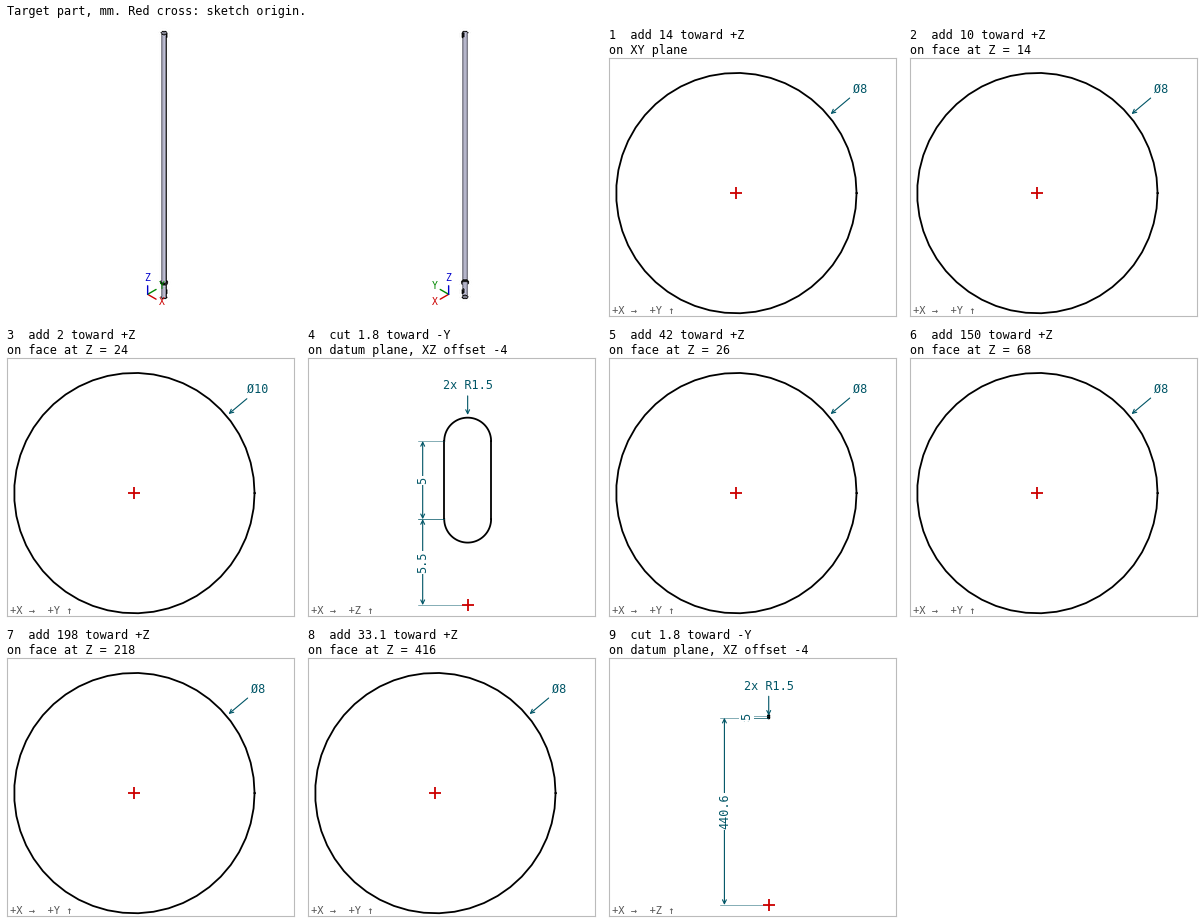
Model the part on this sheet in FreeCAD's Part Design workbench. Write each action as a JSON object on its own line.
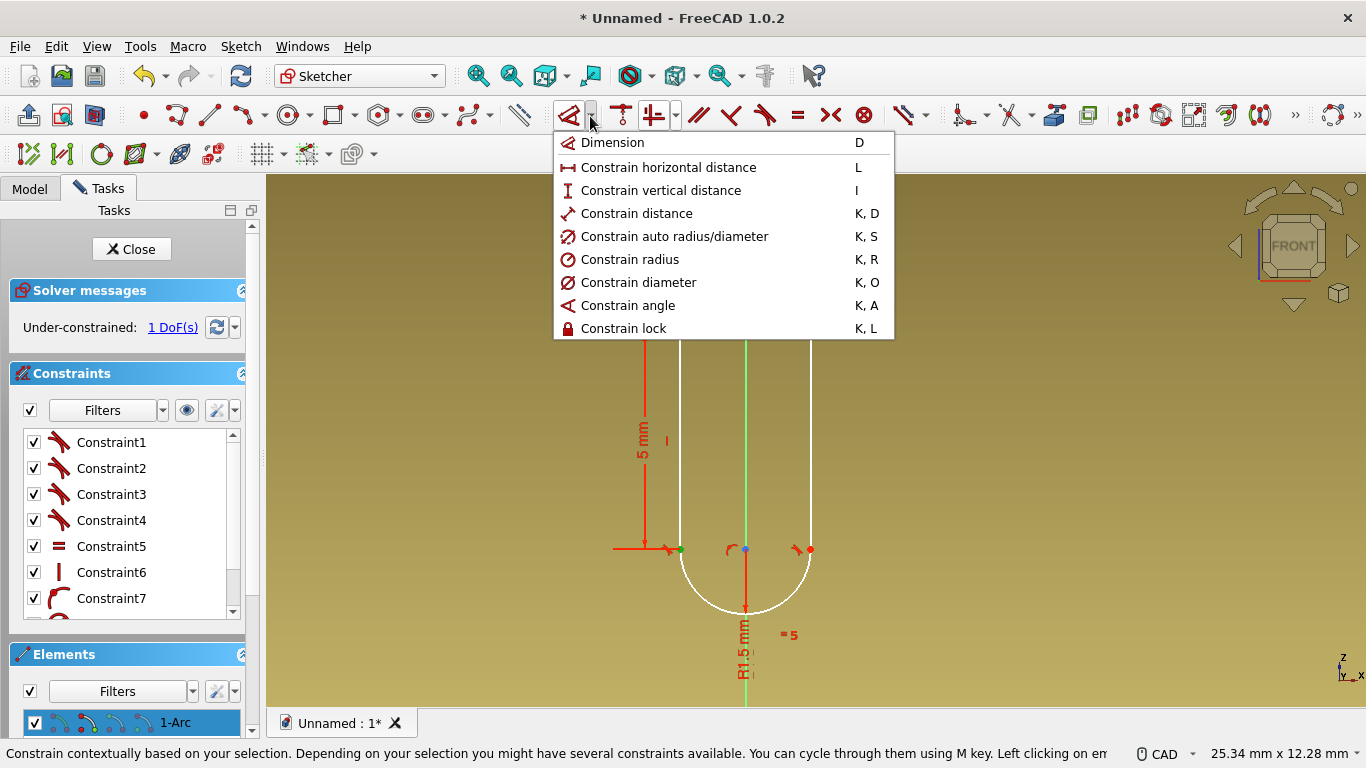
{"action": "left_click", "coordinate": [724, 190]}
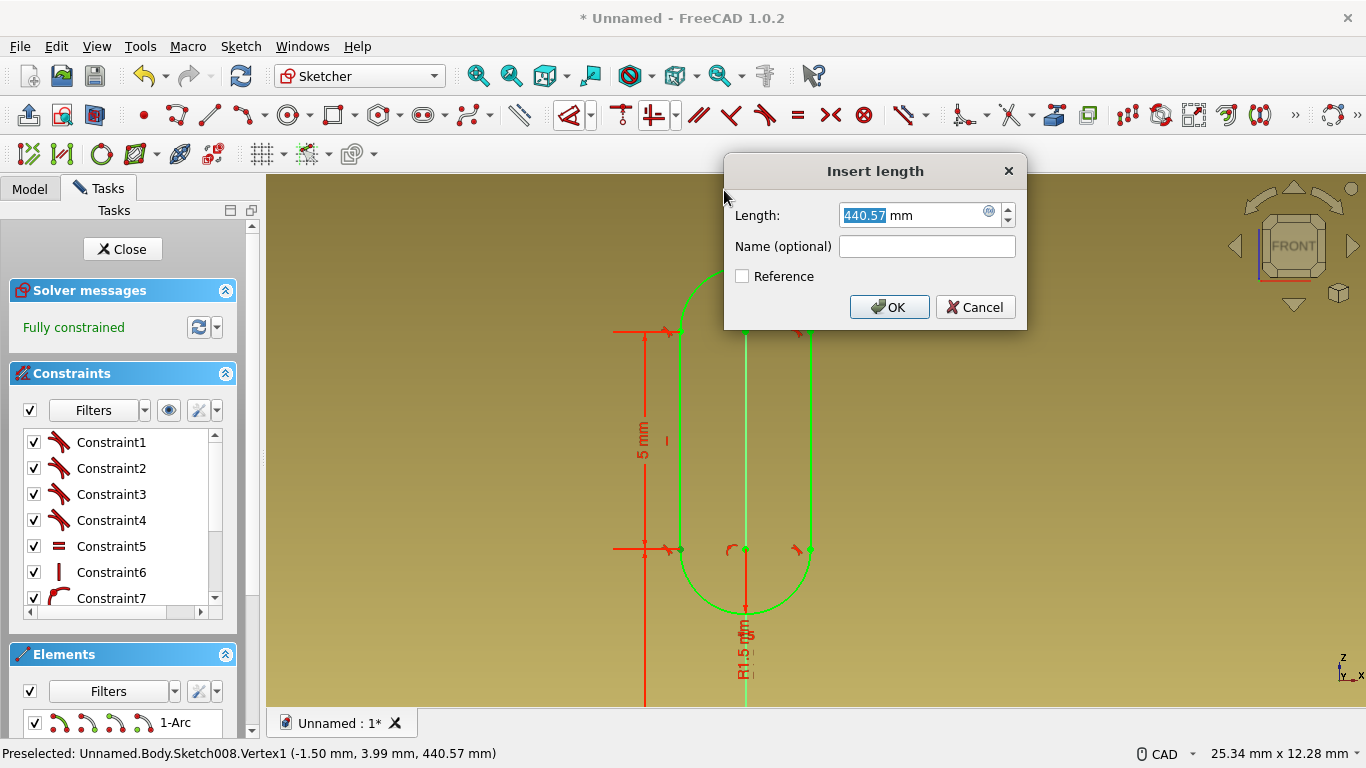
{"action": "type", "text": "440.6"}
{"action": "key", "text": "Return"}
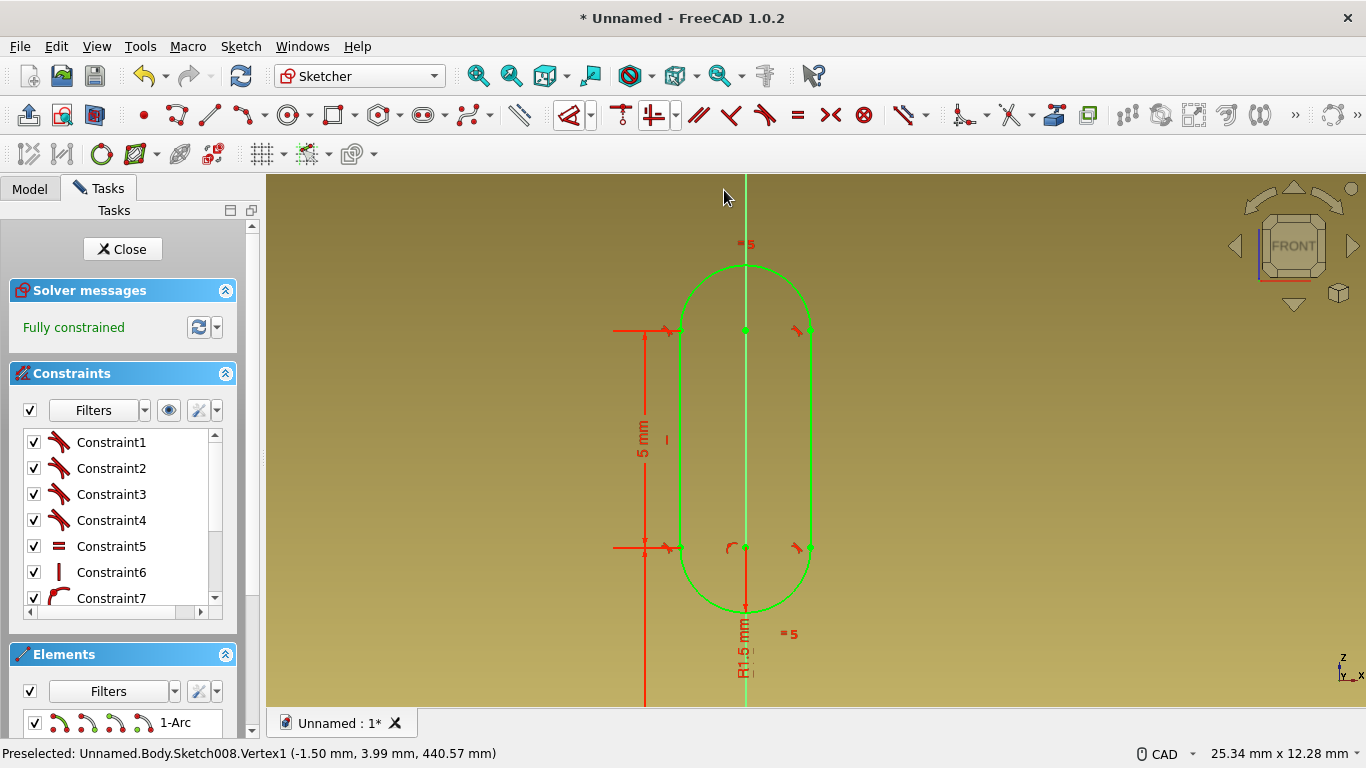
{"action": "left_click", "coordinate": [123, 249]}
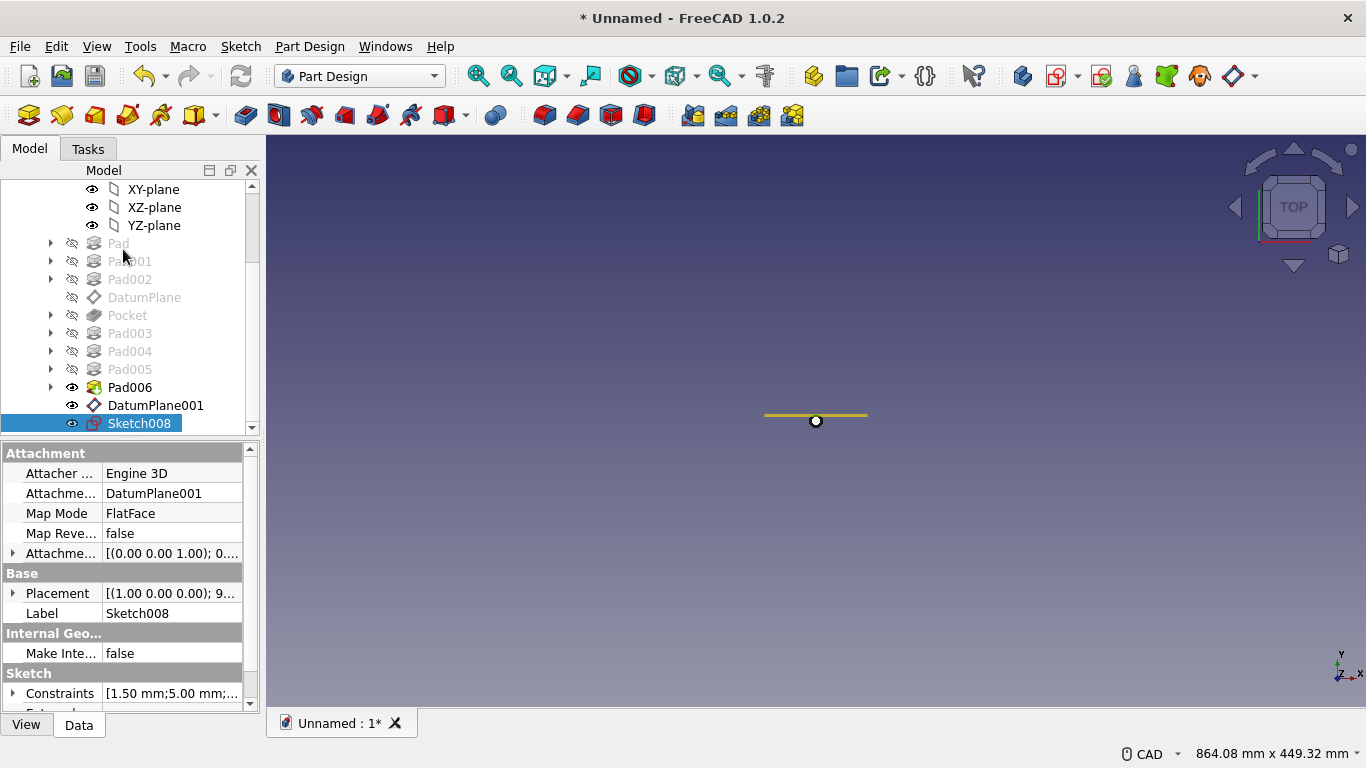
{"action": "left_click", "coordinate": [246, 116]}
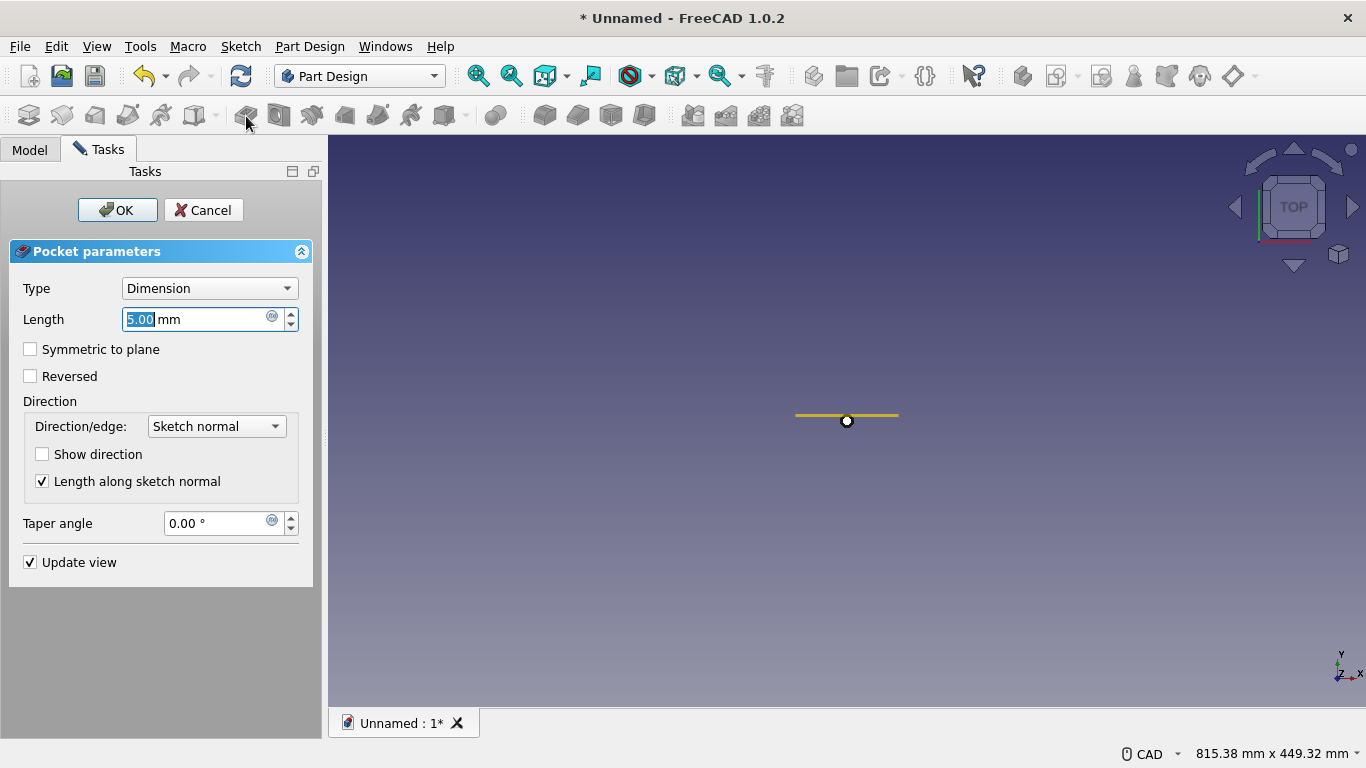
{"action": "type", "text": "1.8"}
{"action": "key", "text": "Tab"}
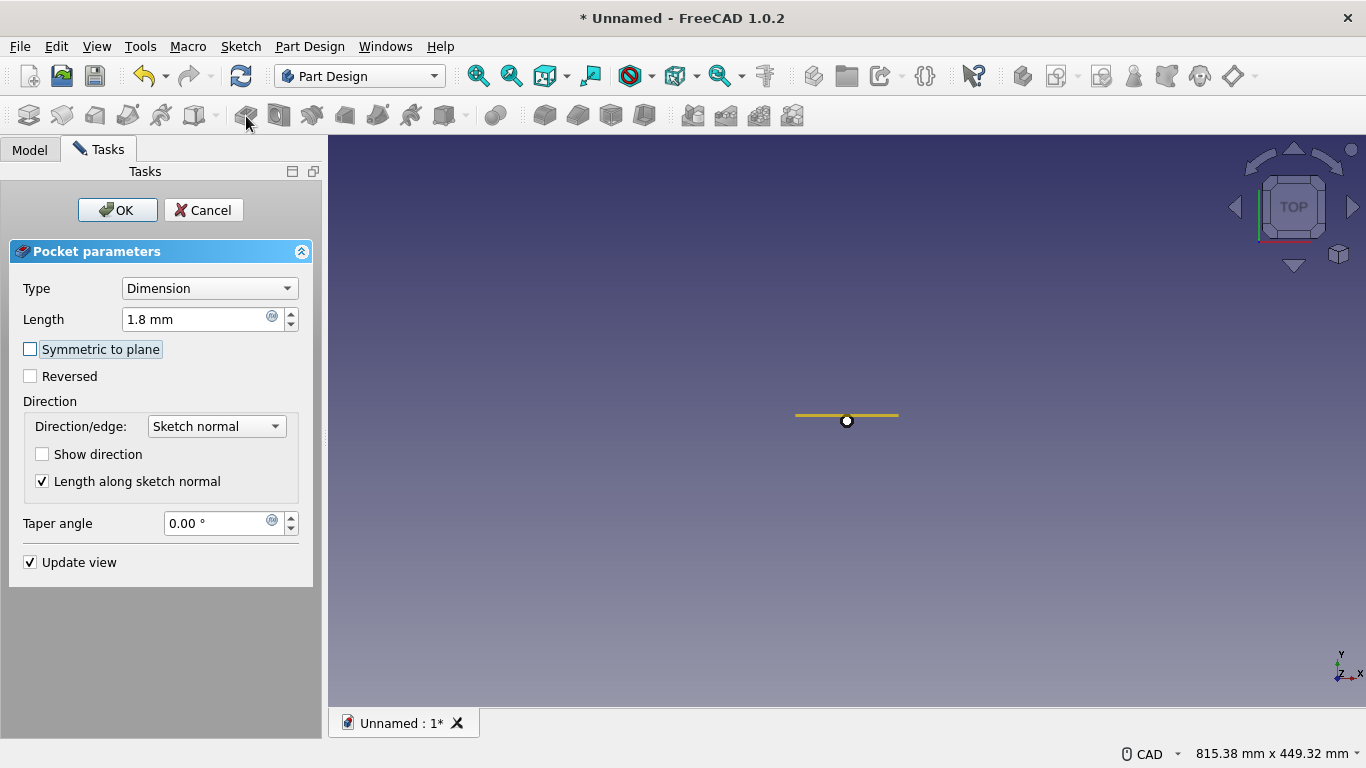
{"action": "left_click", "coordinate": [31, 376]}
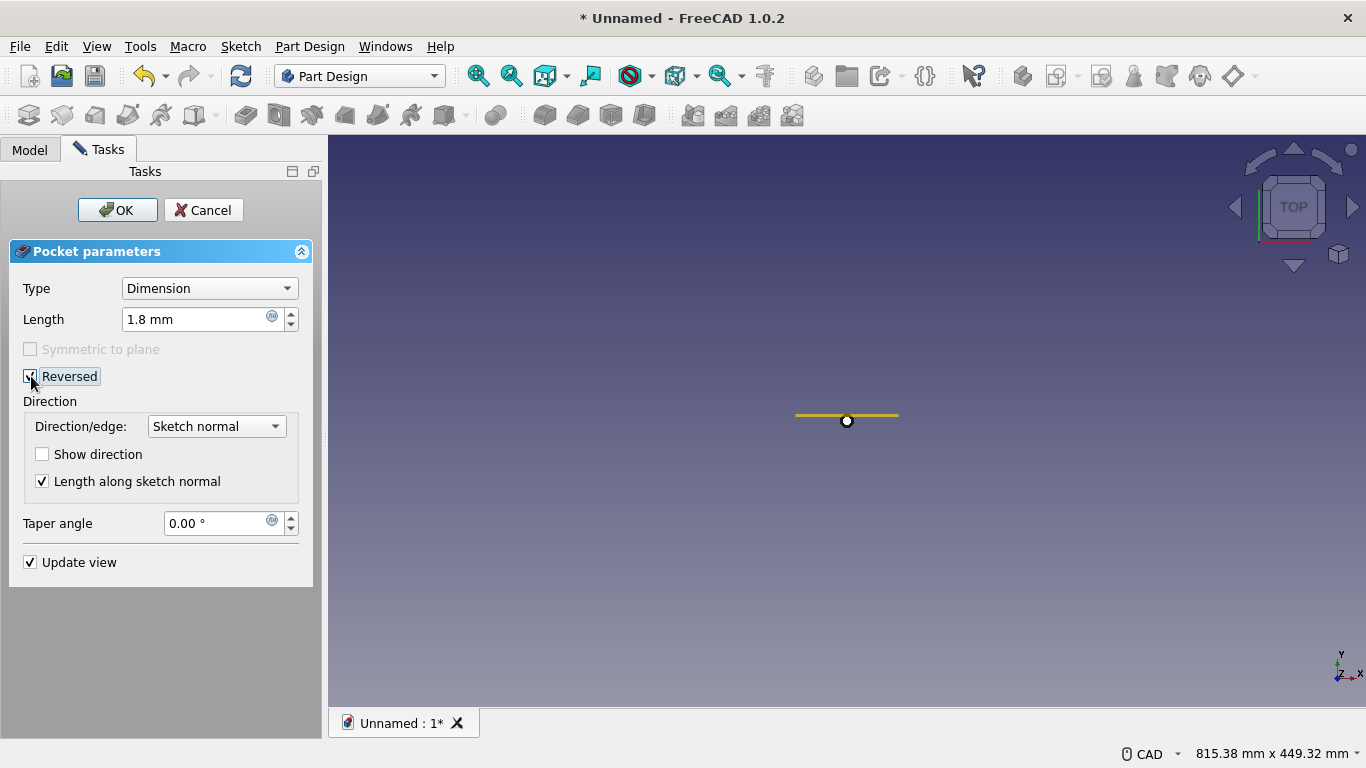
{"action": "left_click", "coordinate": [118, 210]}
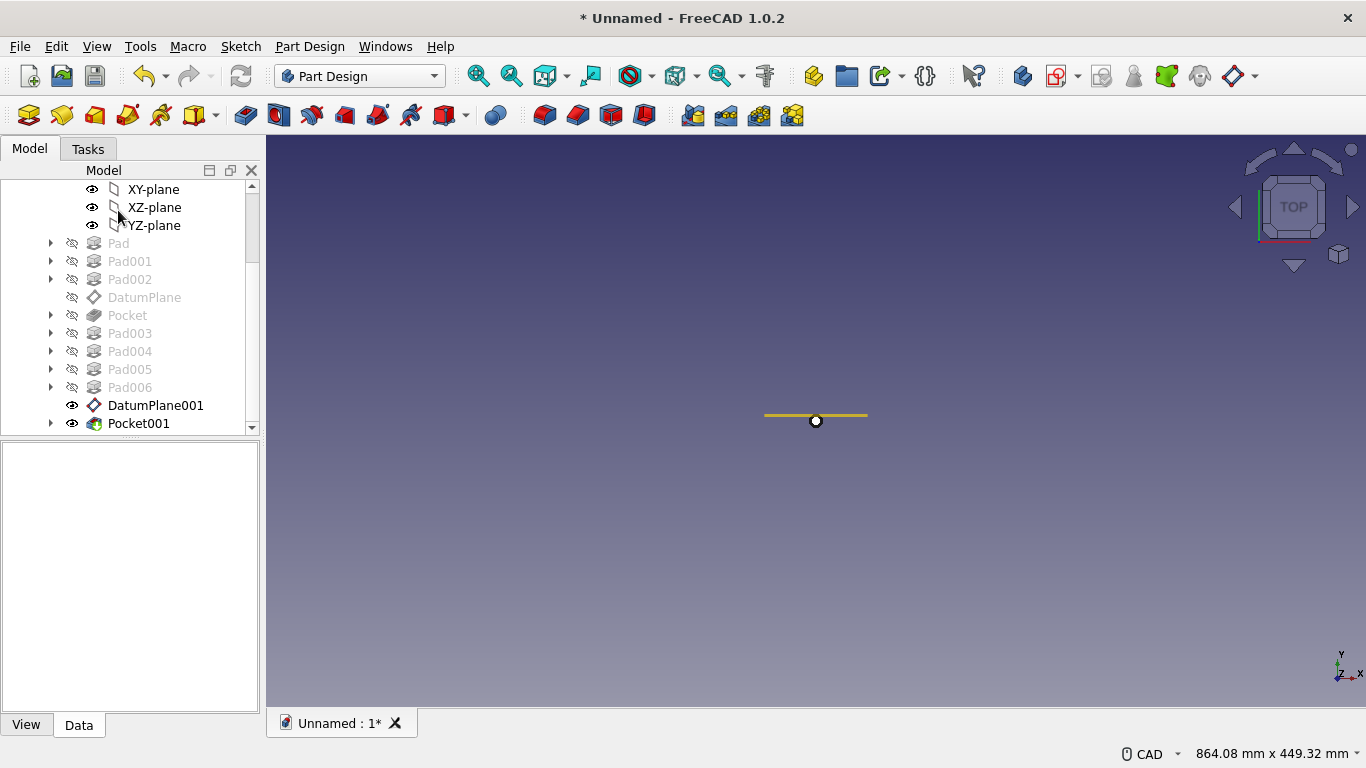
{"action": "left_click", "coordinate": [117, 405]}
{"action": "key", "text": "space"}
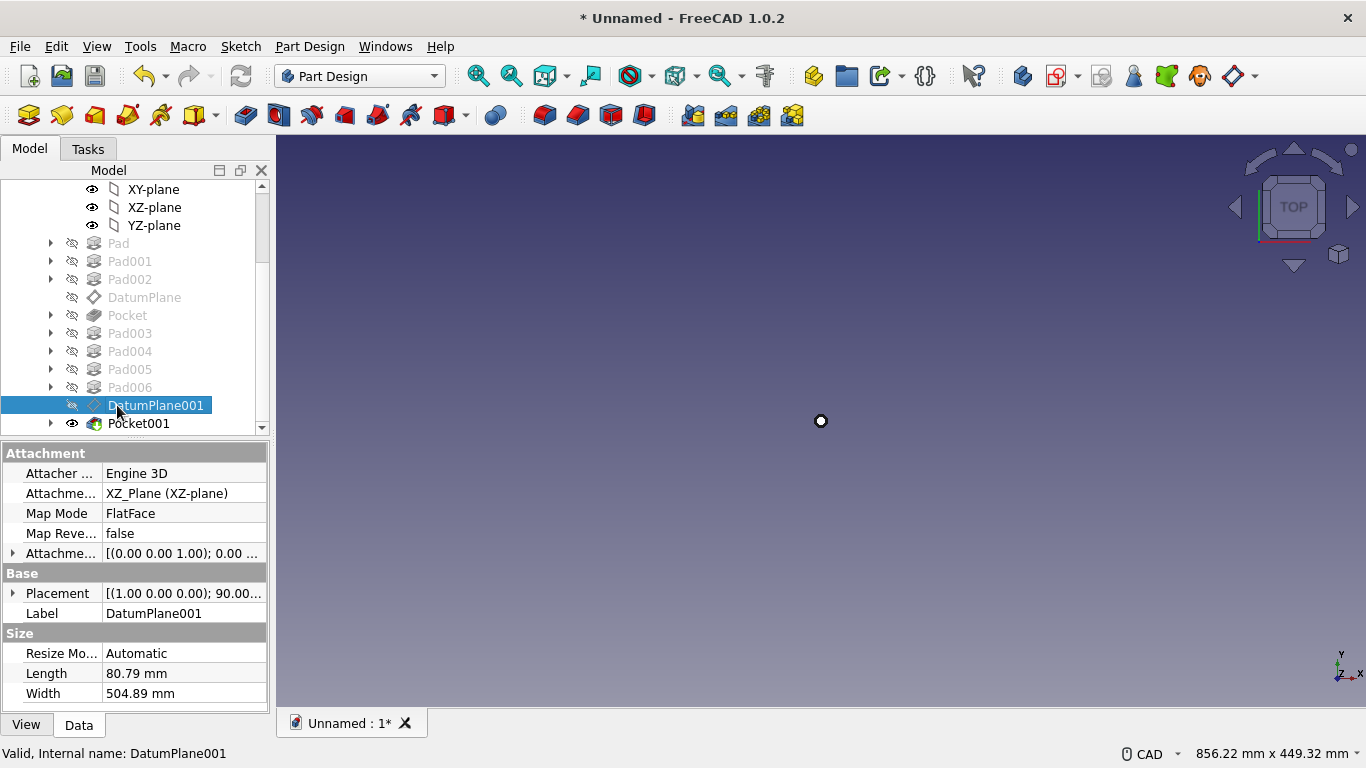
{"action": "key", "text": "0"}